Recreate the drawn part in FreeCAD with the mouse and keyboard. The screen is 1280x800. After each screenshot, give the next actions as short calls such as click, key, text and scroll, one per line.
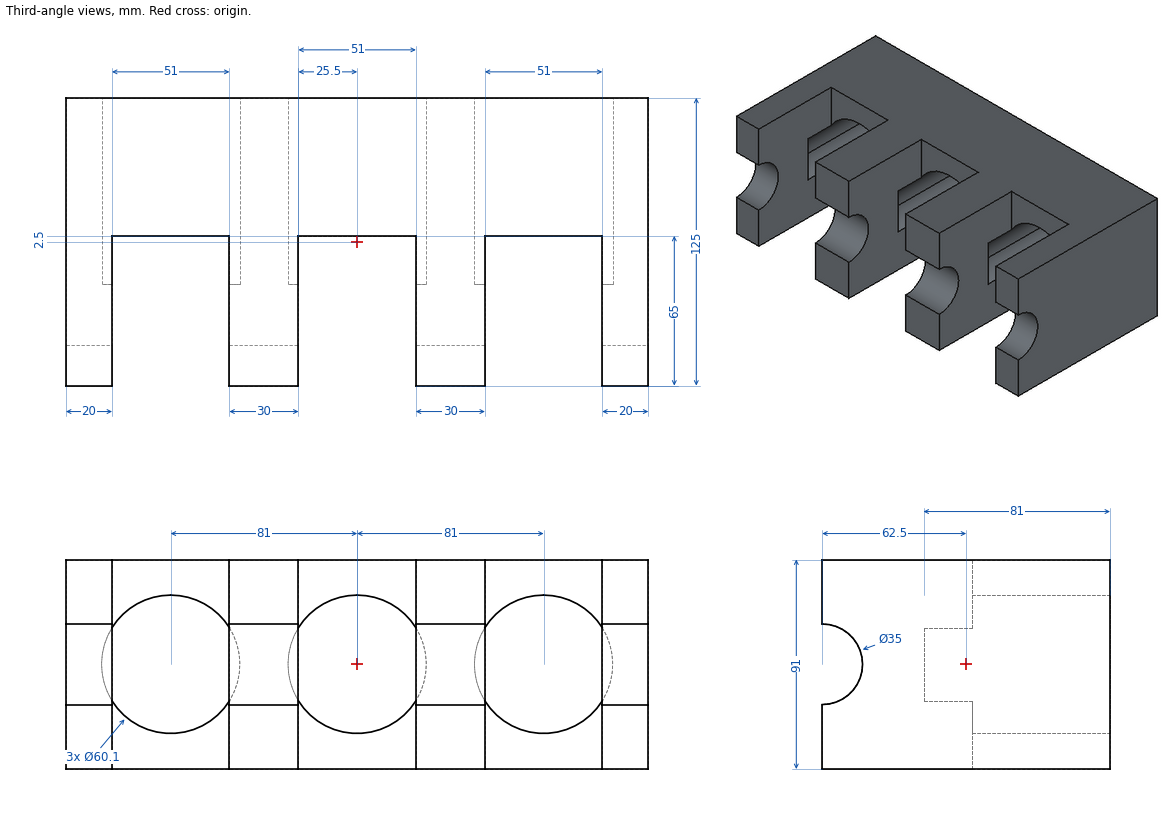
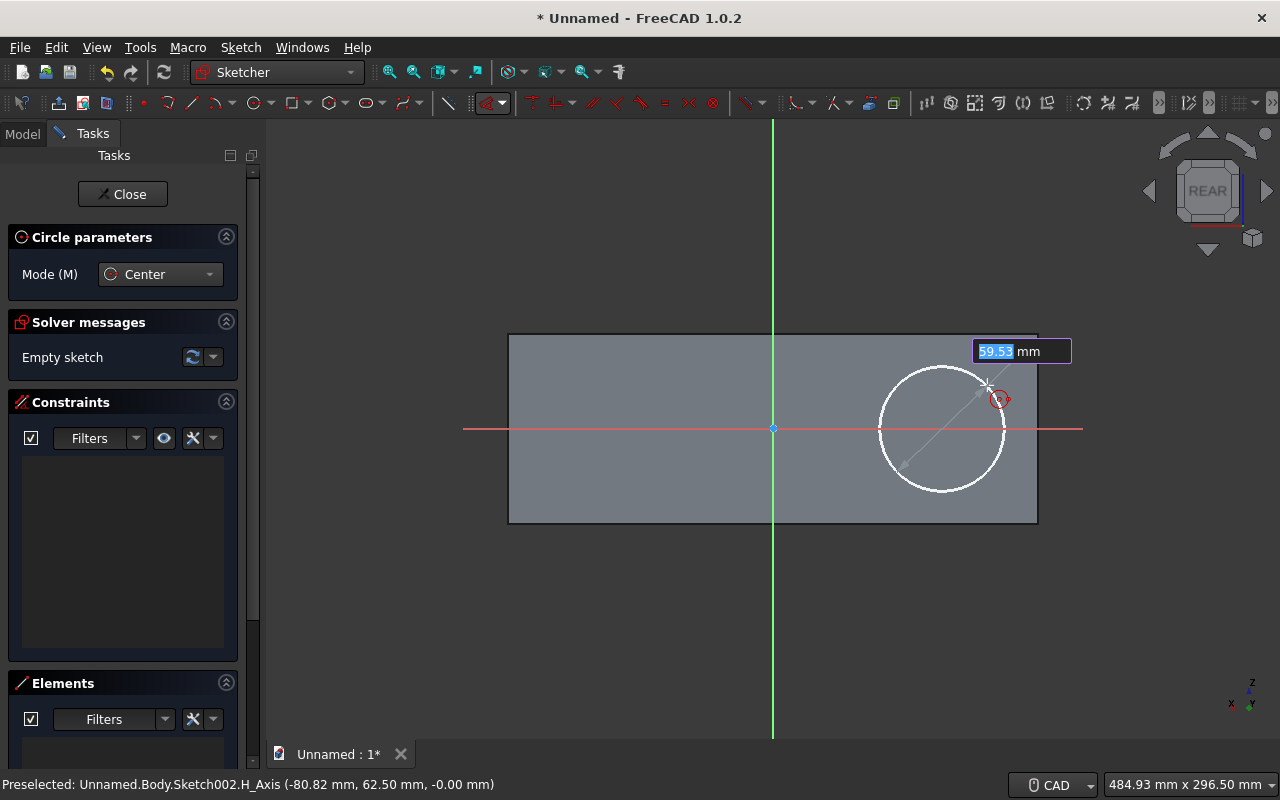
text(60.1)
key(Return)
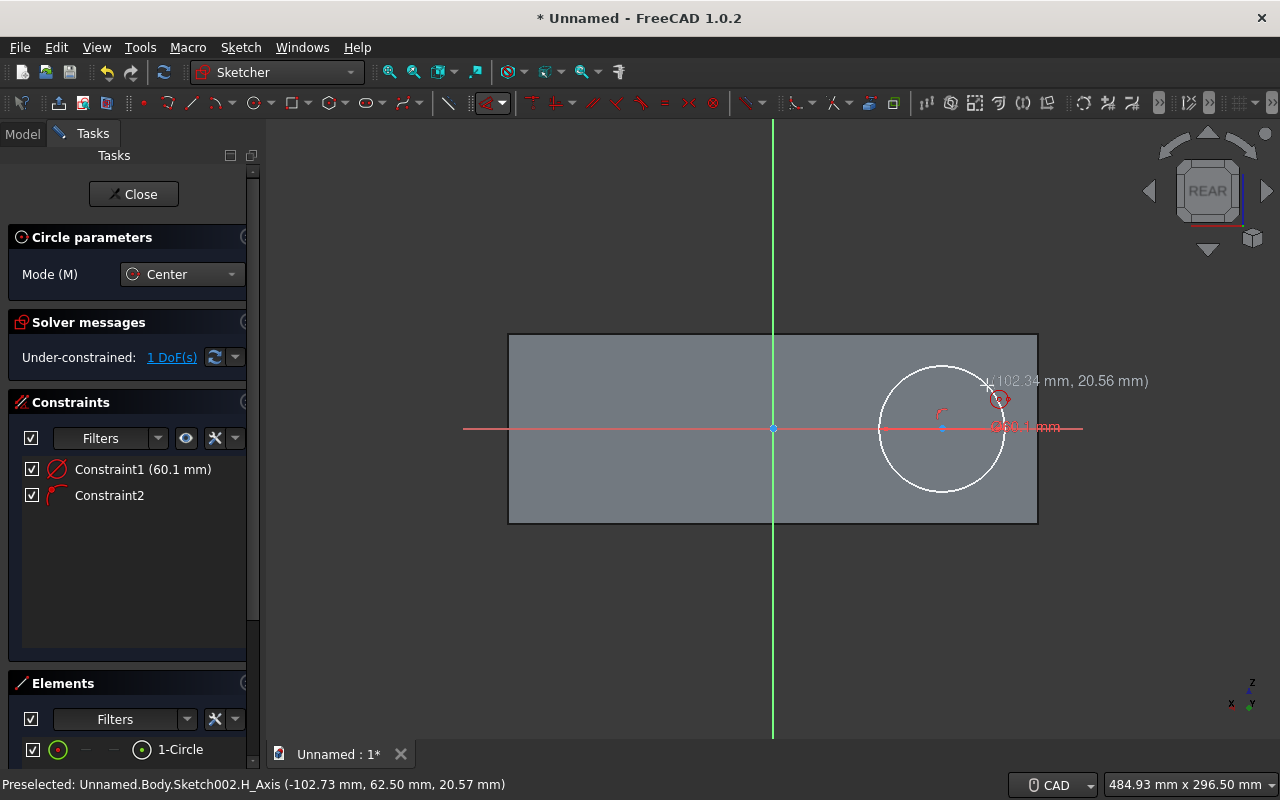
click(773, 429)
move(817, 385)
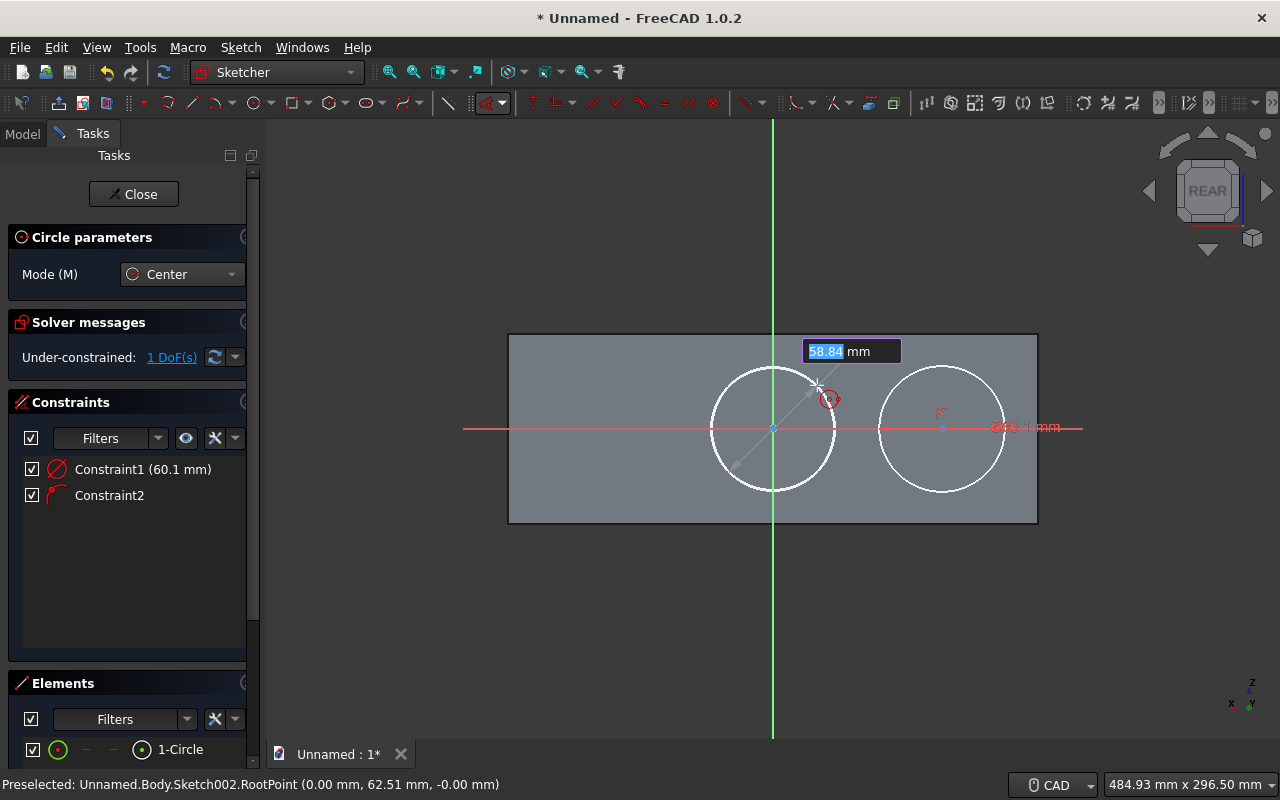
text(60.1)
key(Return)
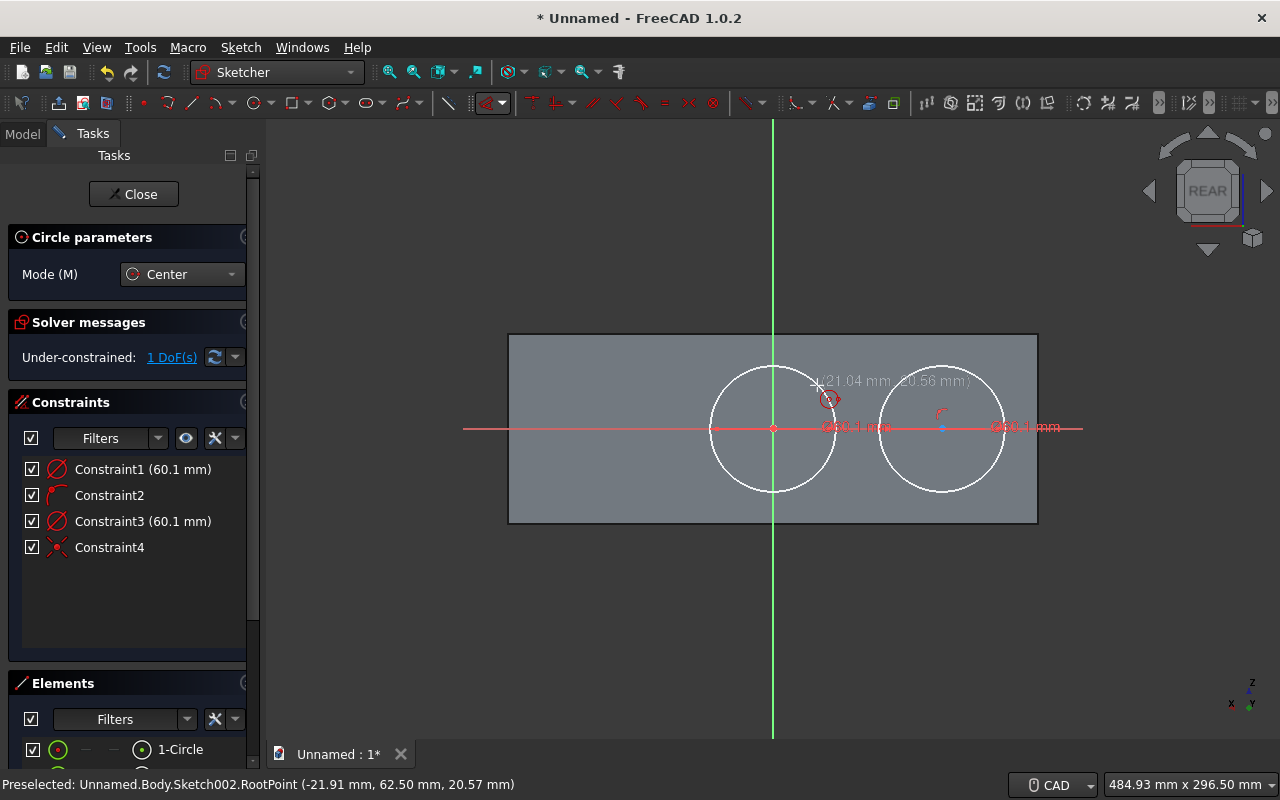
click(604, 429)
move(648, 385)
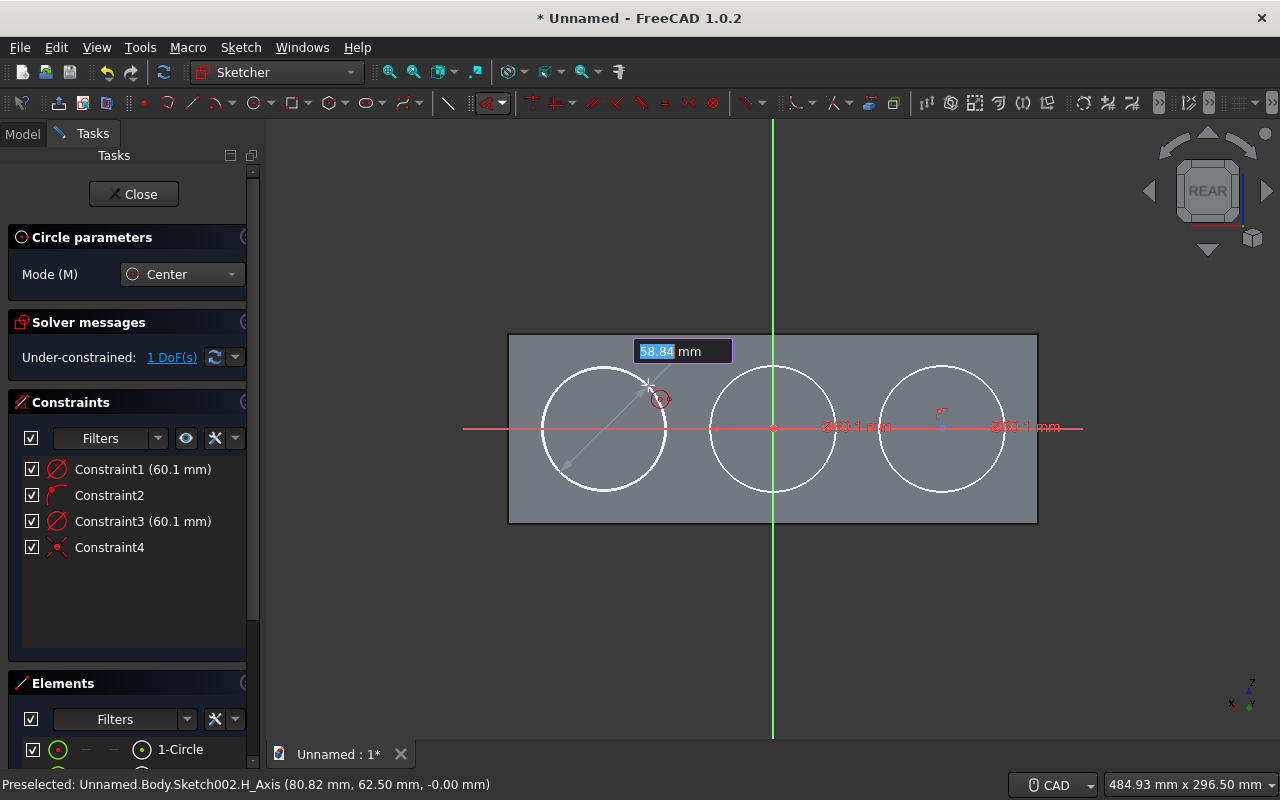
text(60.1)
key(Return)
key(Escape)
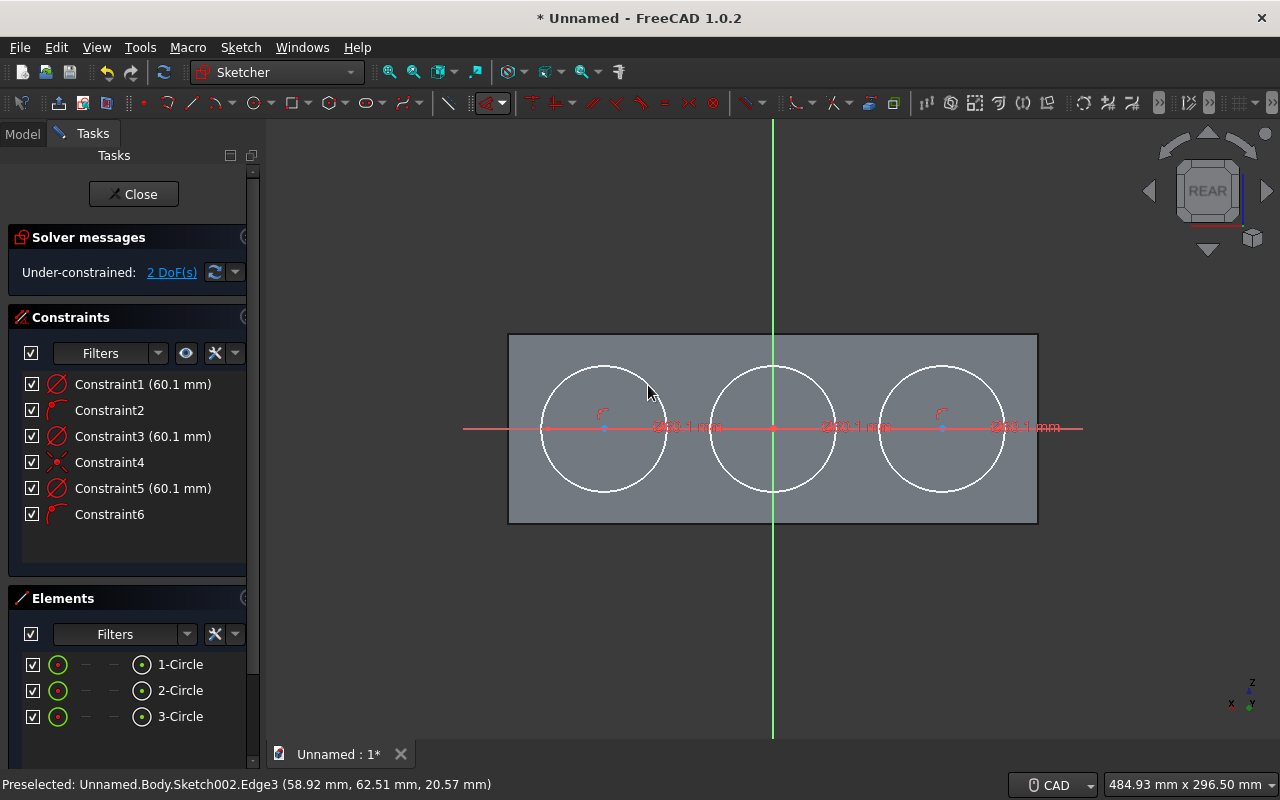
click(942, 429)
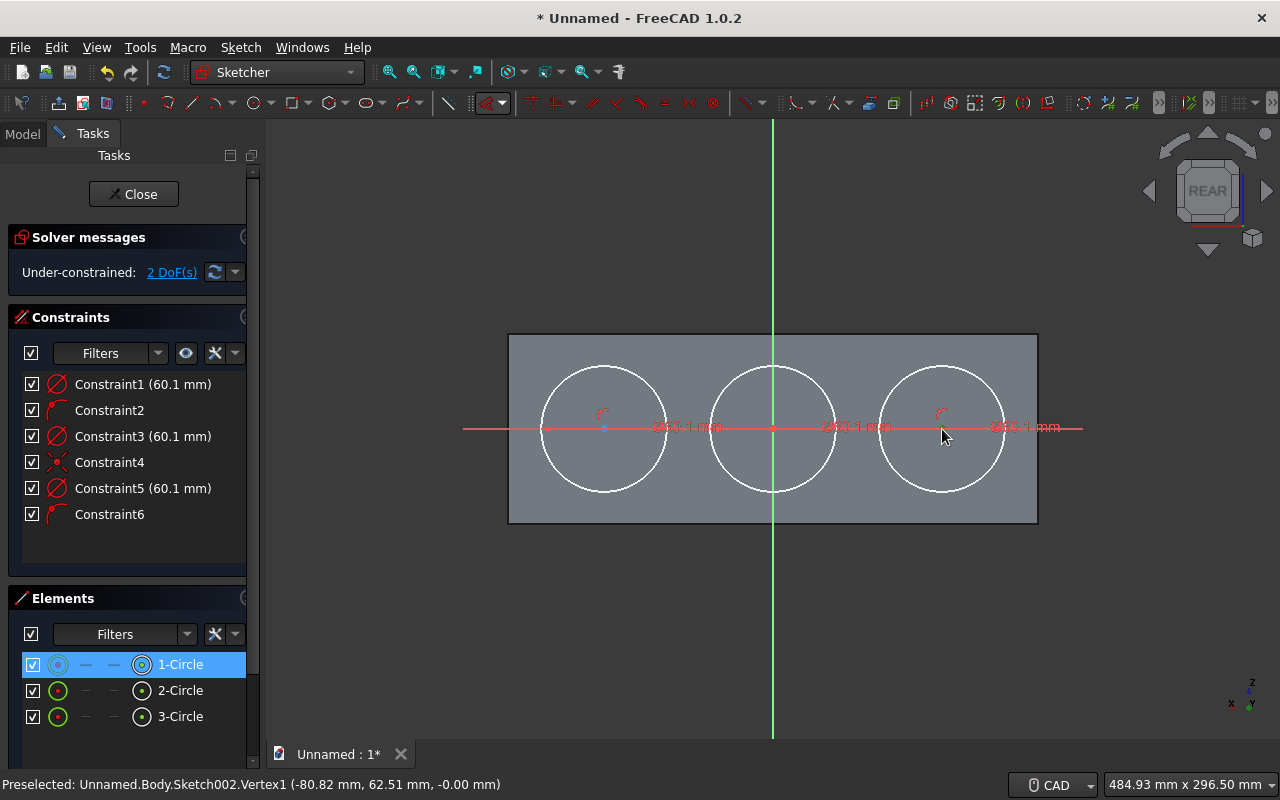
key(l)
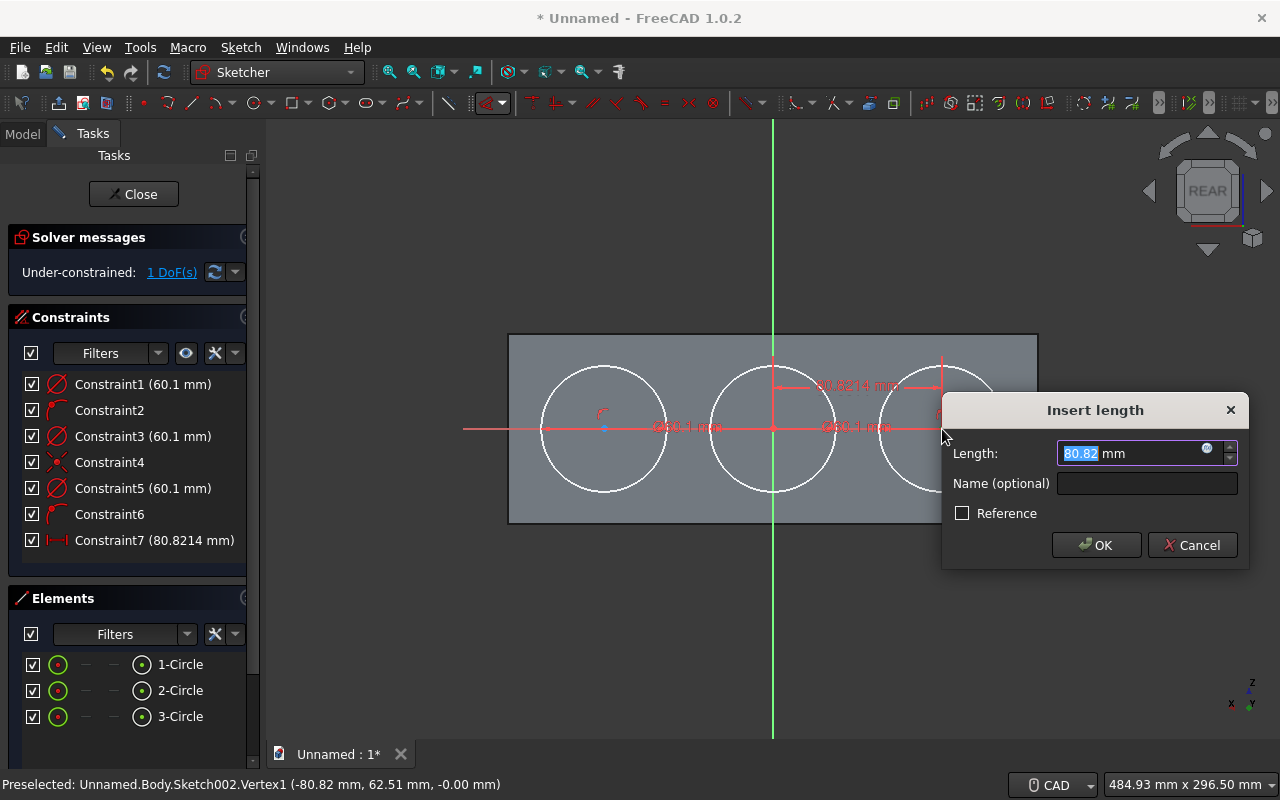
text(81)
key(Return)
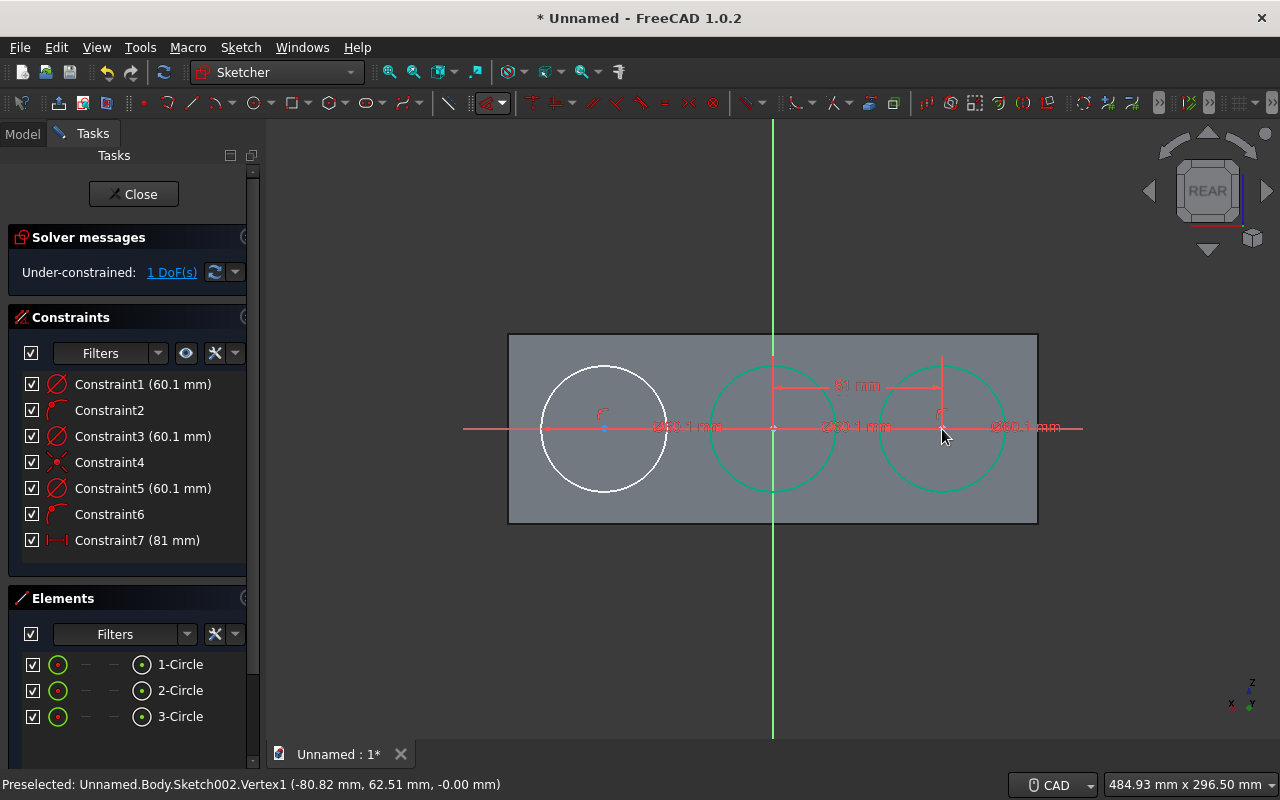
click(604, 429)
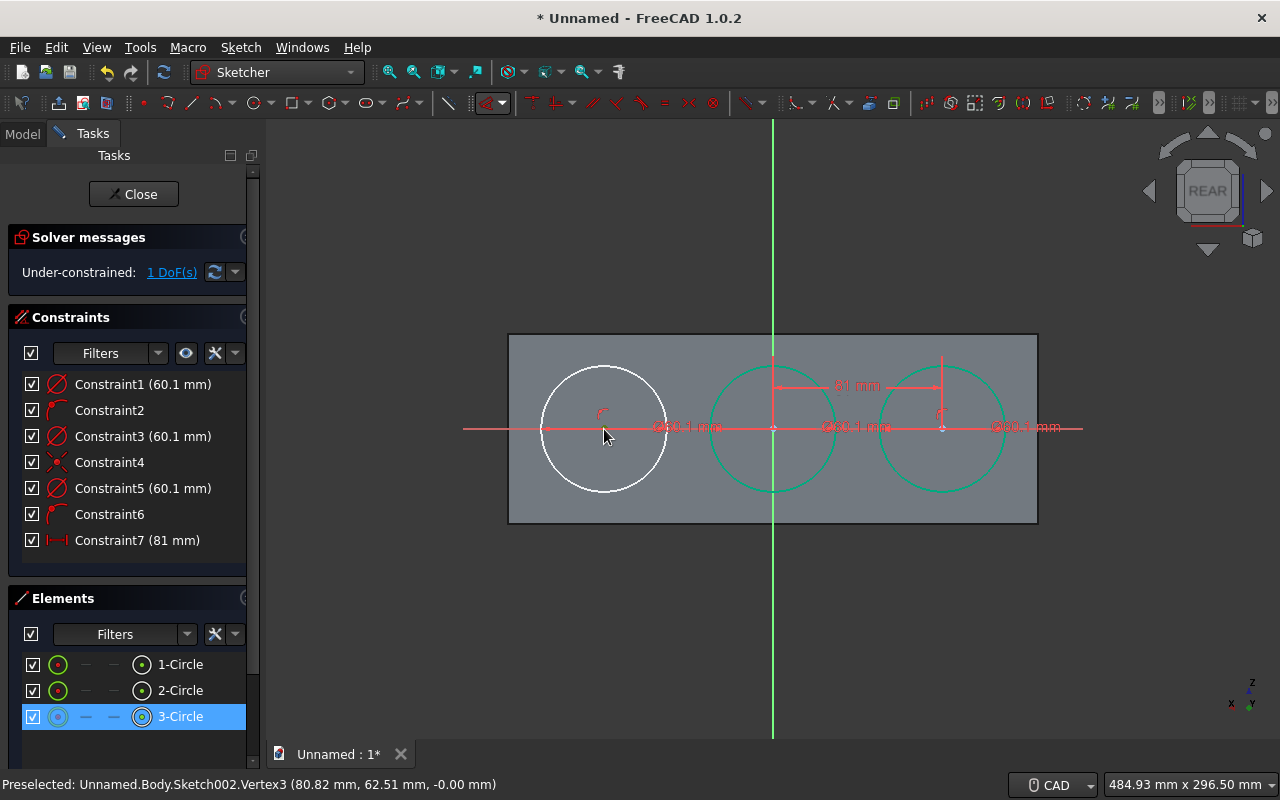
key(l)